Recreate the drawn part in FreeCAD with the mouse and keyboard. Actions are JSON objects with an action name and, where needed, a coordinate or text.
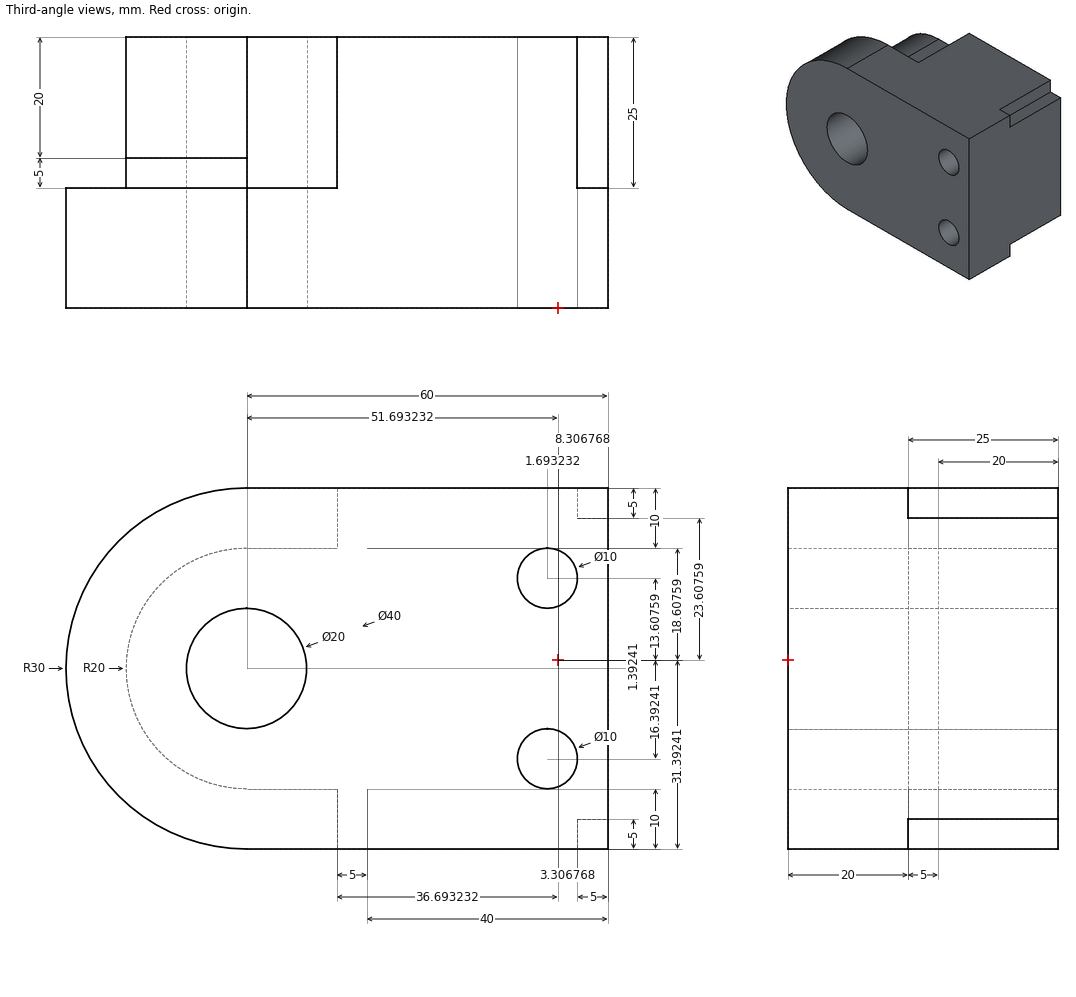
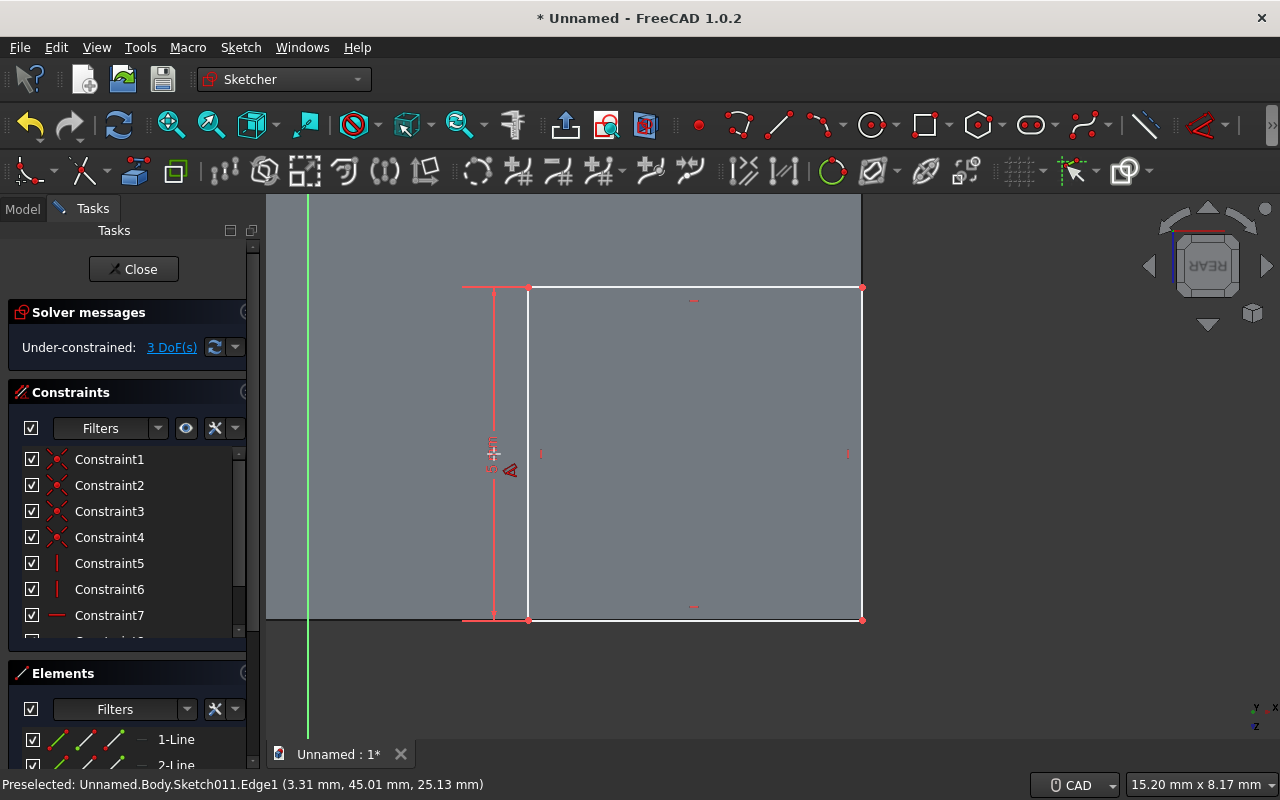
{"action": "left_click", "coordinate": [628, 621]}
{"action": "left_click", "coordinate": [695, 655]}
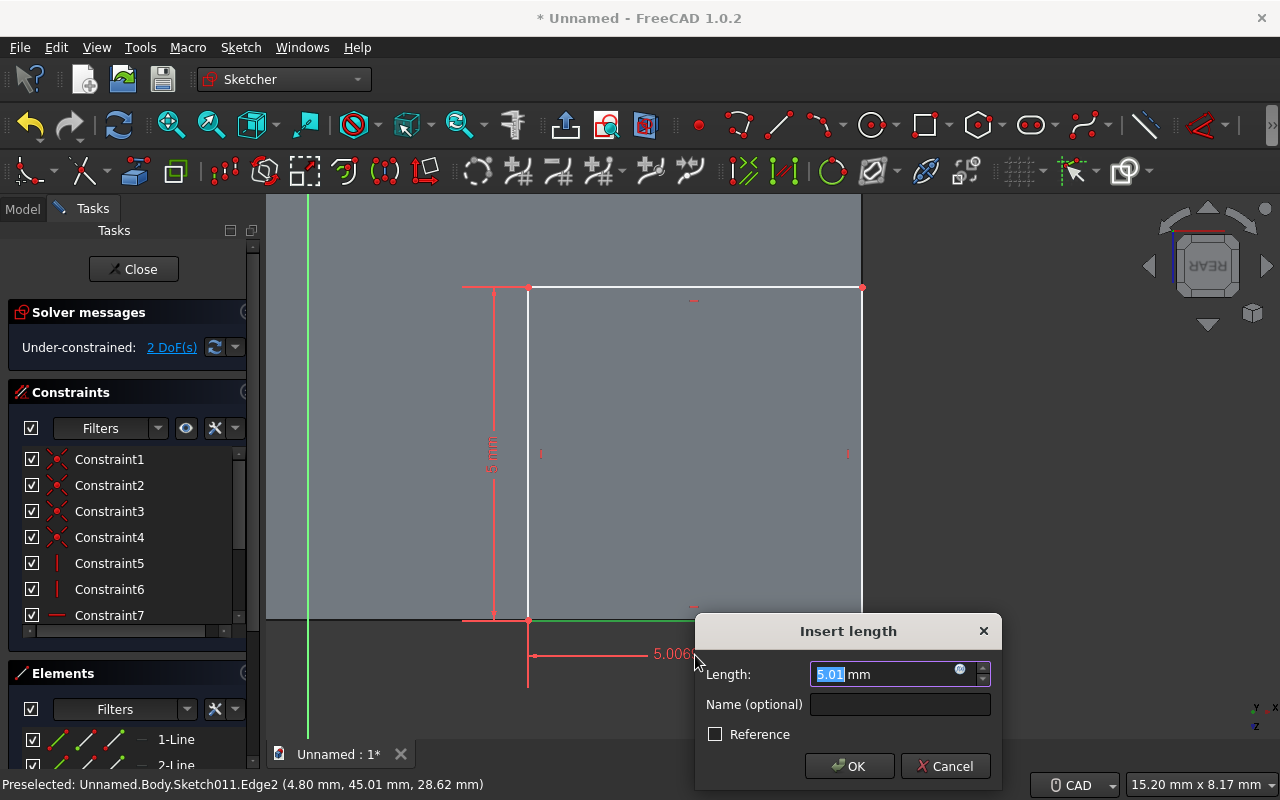
{"action": "type", "text": "5"}
{"action": "key", "text": "Return"}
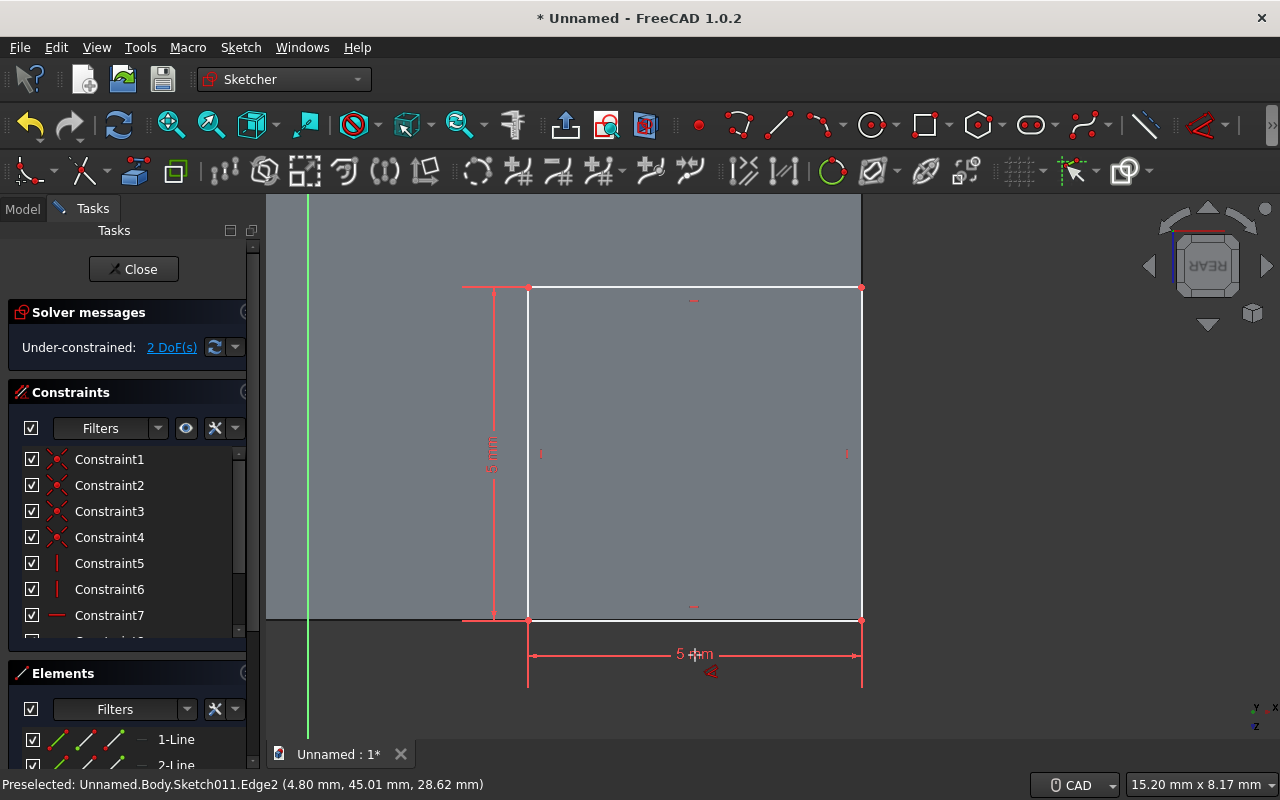
{"action": "left_click", "coordinate": [528, 287]}
{"action": "left_click", "coordinate": [418, 321]}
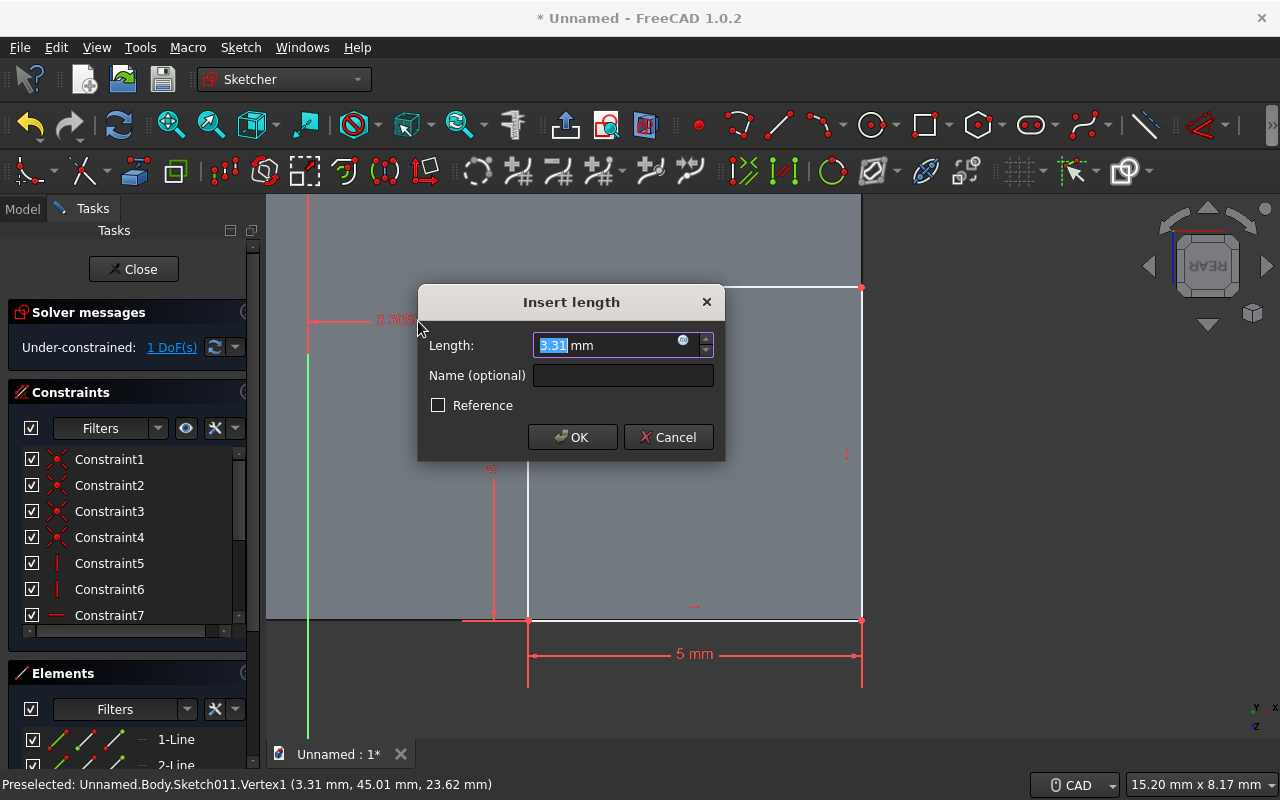
{"action": "type", "text": "3.306768"}
{"action": "key", "text": "Return"}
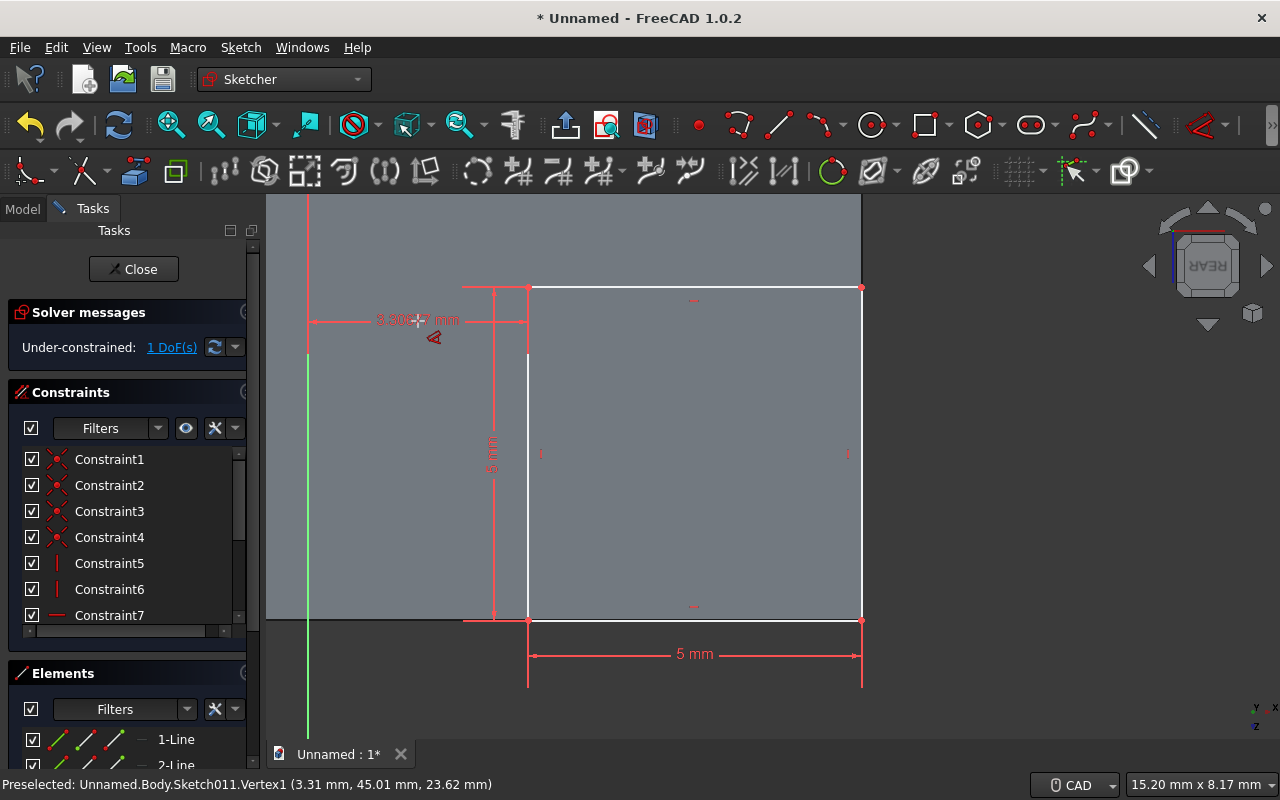
{"action": "left_click", "coordinate": [528, 287]}
{"action": "left_click", "coordinate": [562, 254]}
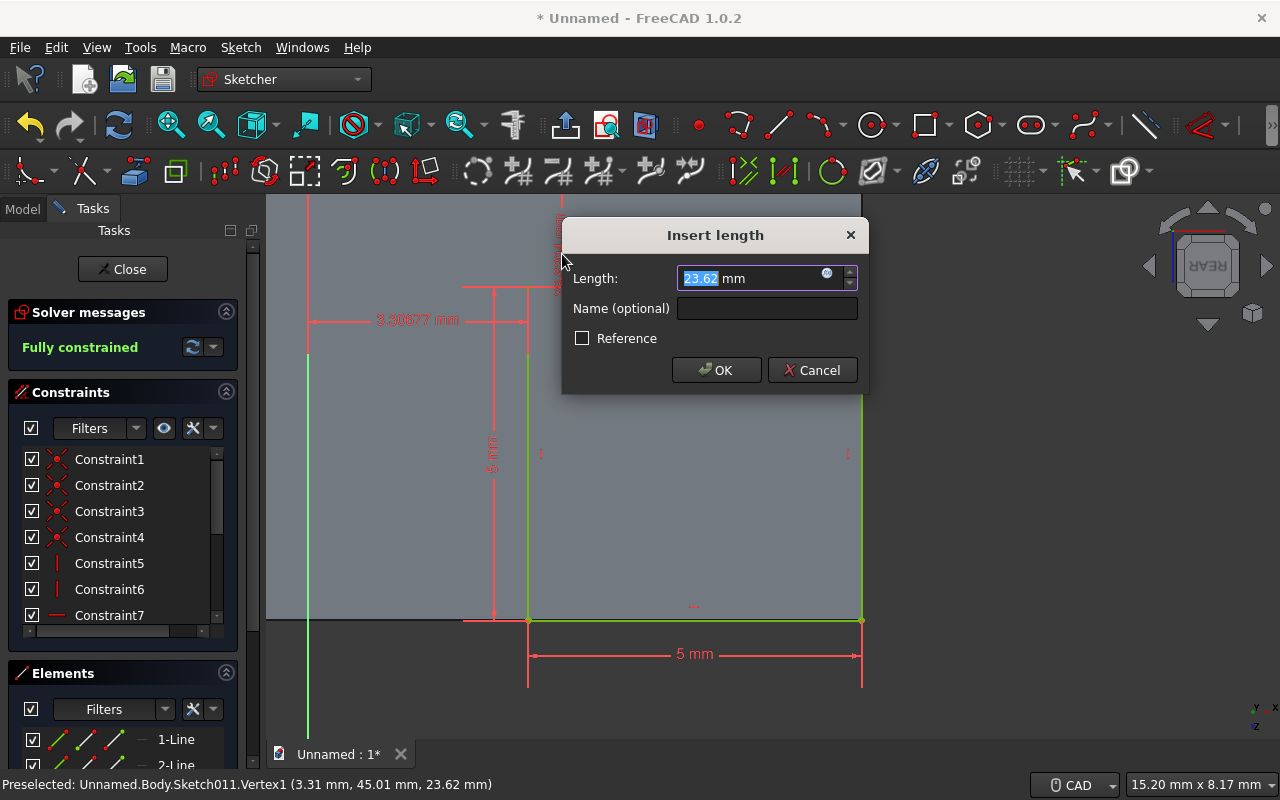
{"action": "type", "text": "23.60759"}
{"action": "key", "text": "Return"}
{"action": "key", "text": "Escape"}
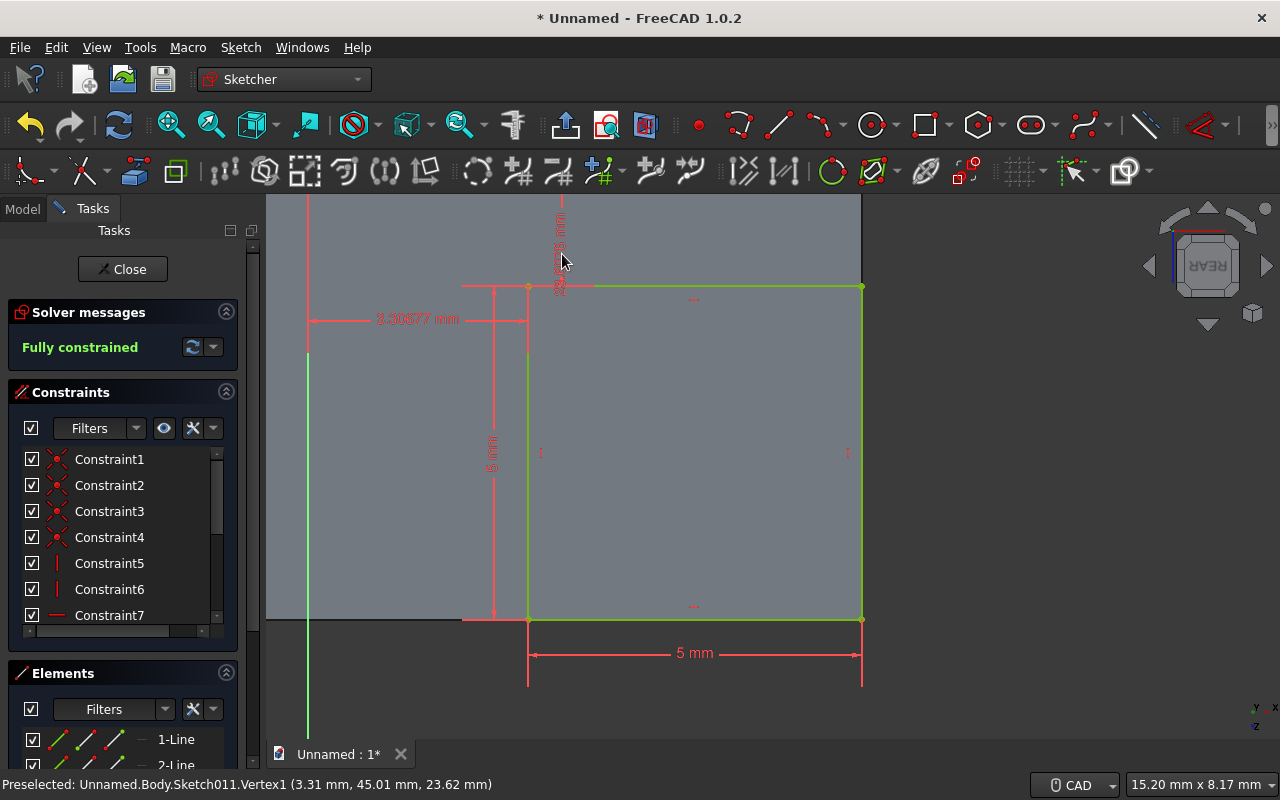
{"action": "left_click", "coordinate": [123, 269]}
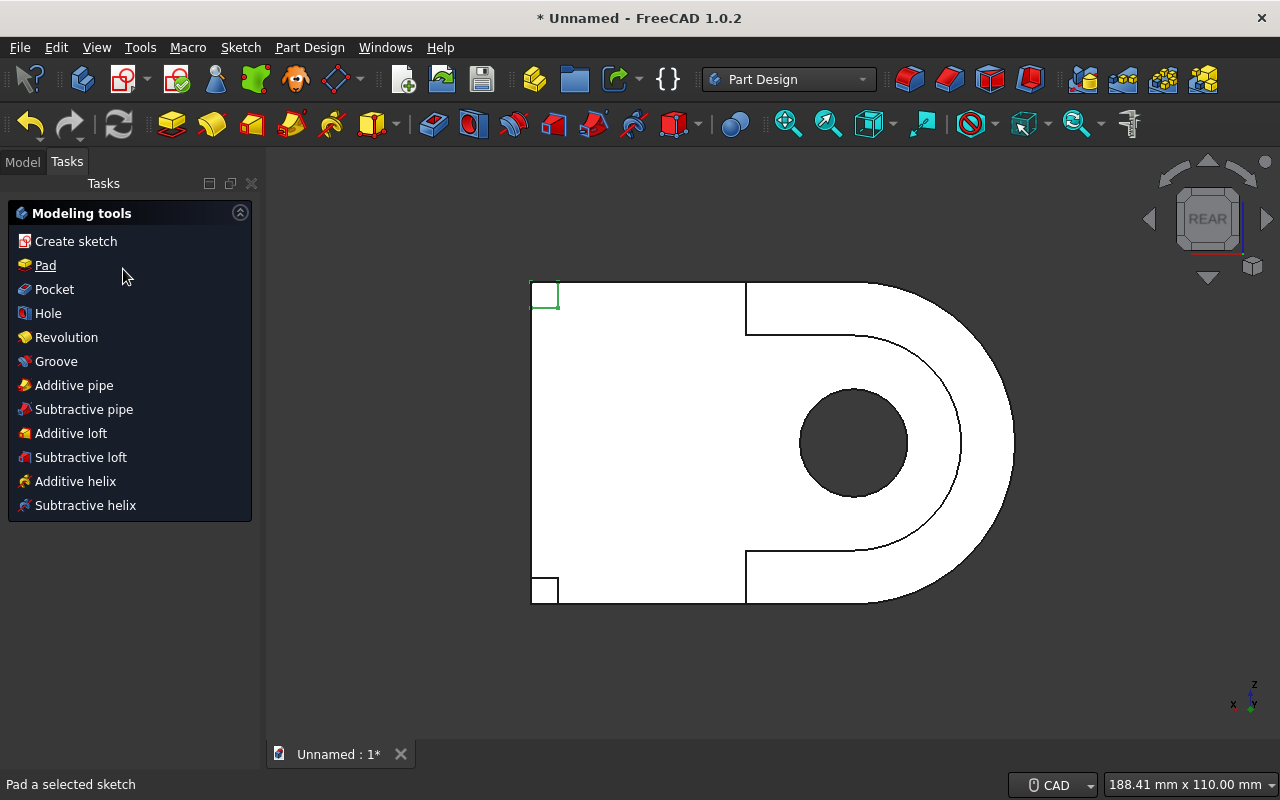
{"action": "left_click", "coordinate": [434, 124]}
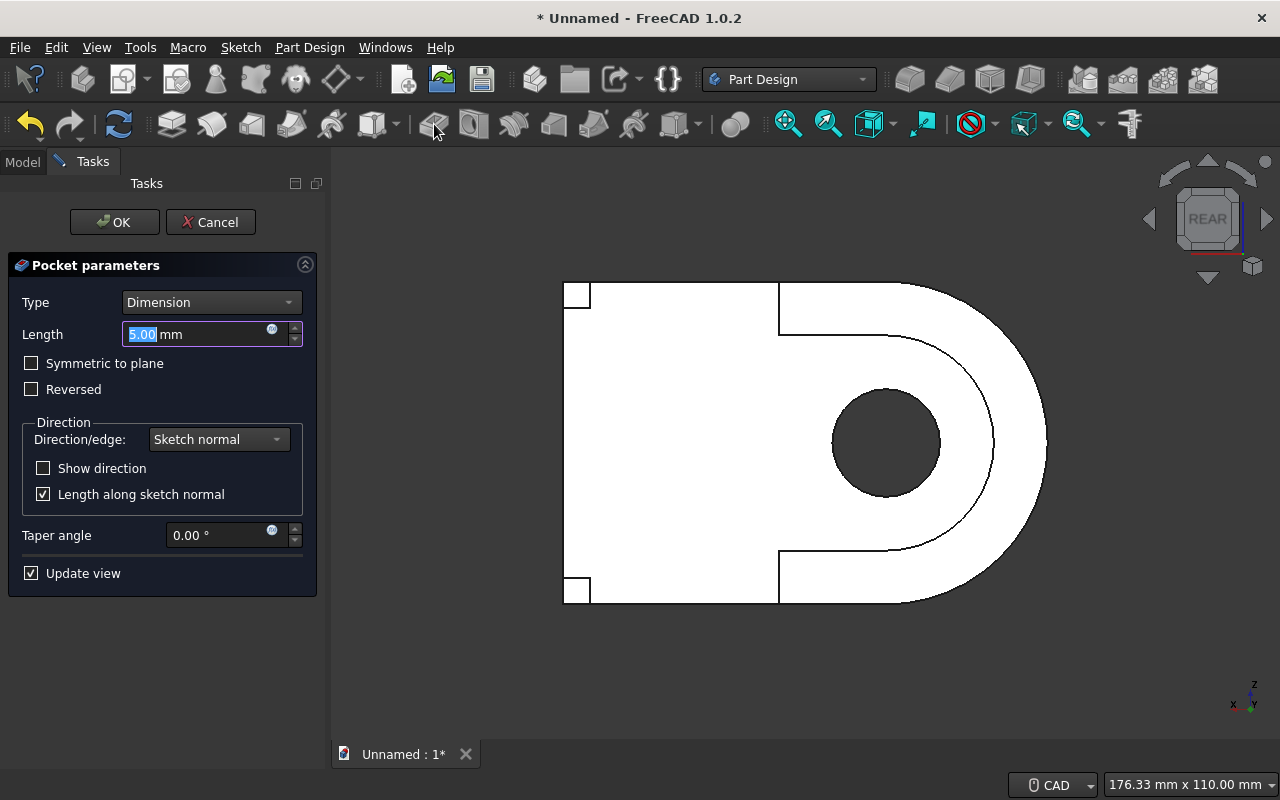
{"action": "type", "text": "25"}
{"action": "key", "text": "Tab"}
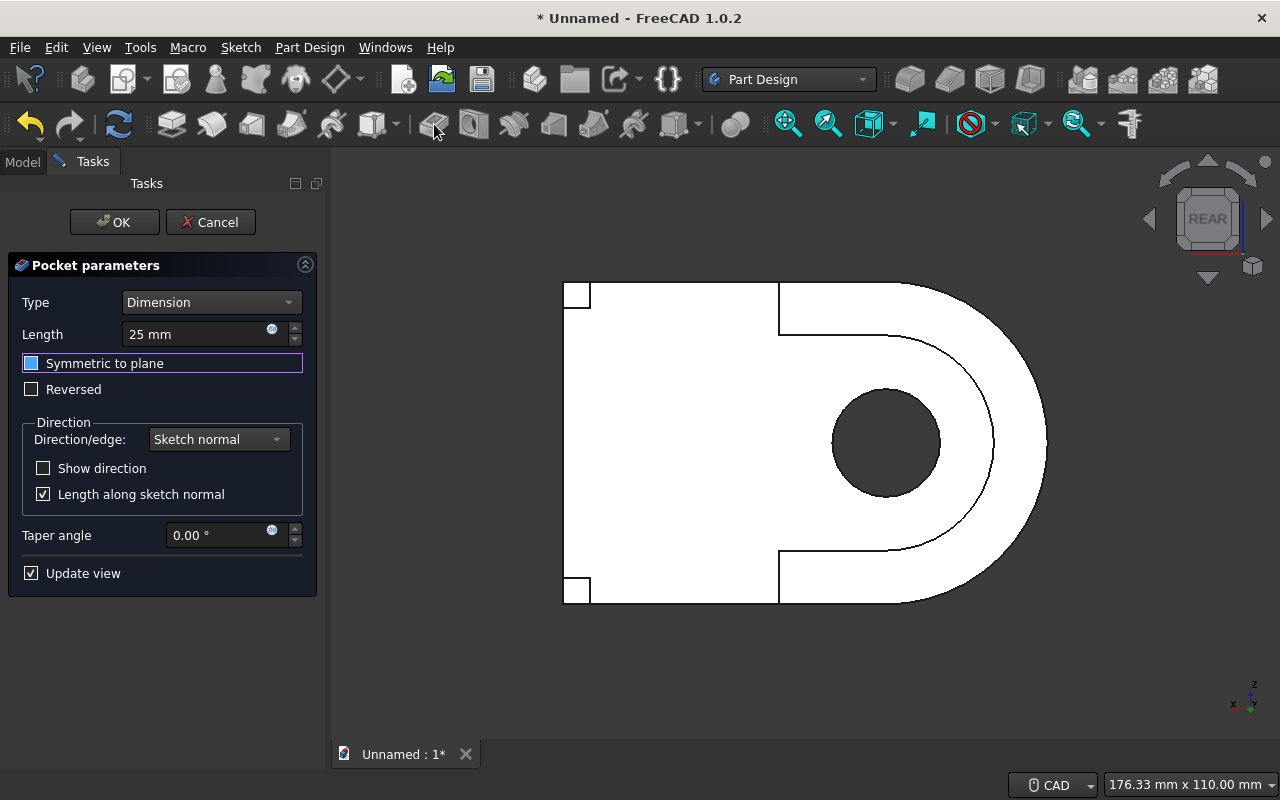
{"action": "left_click", "coordinate": [115, 222]}